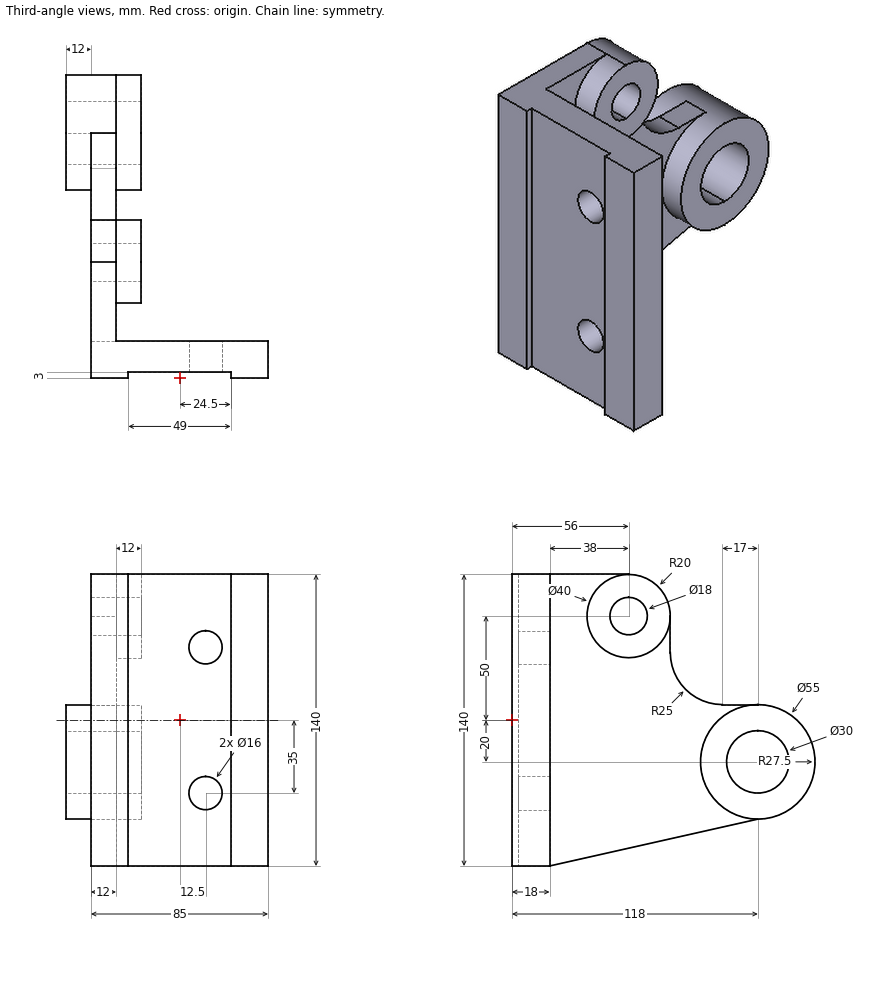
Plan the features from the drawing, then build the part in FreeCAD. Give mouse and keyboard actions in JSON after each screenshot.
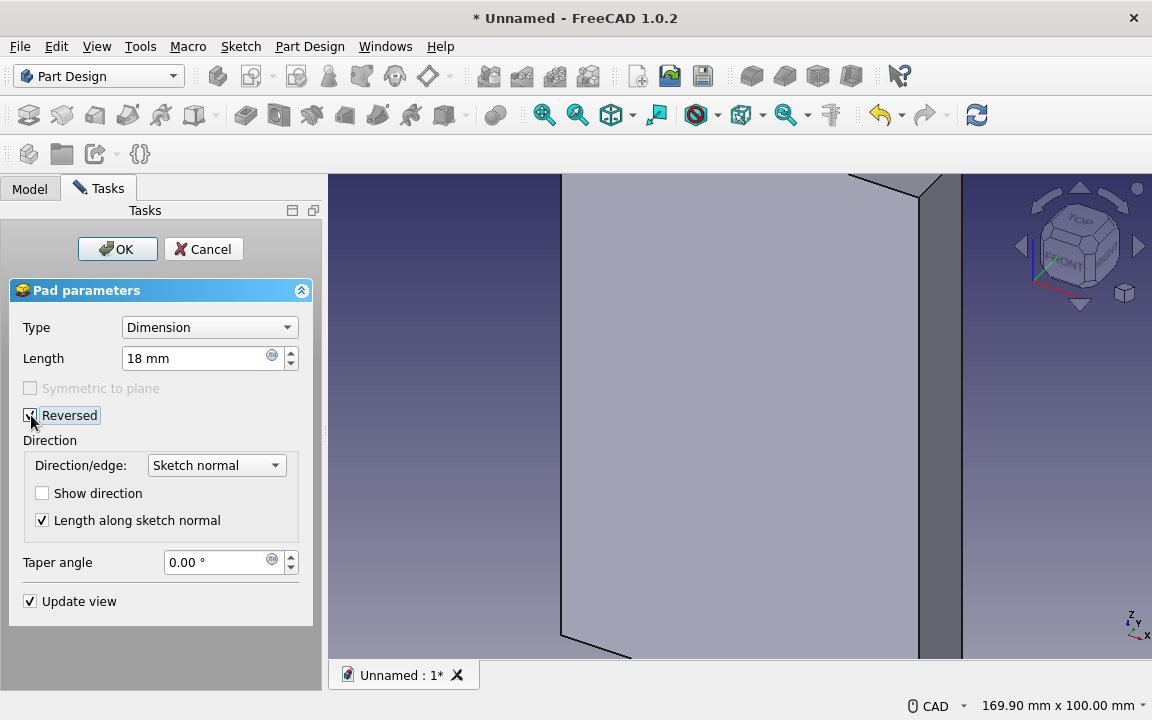
{"action": "left_click", "coordinate": [118, 249]}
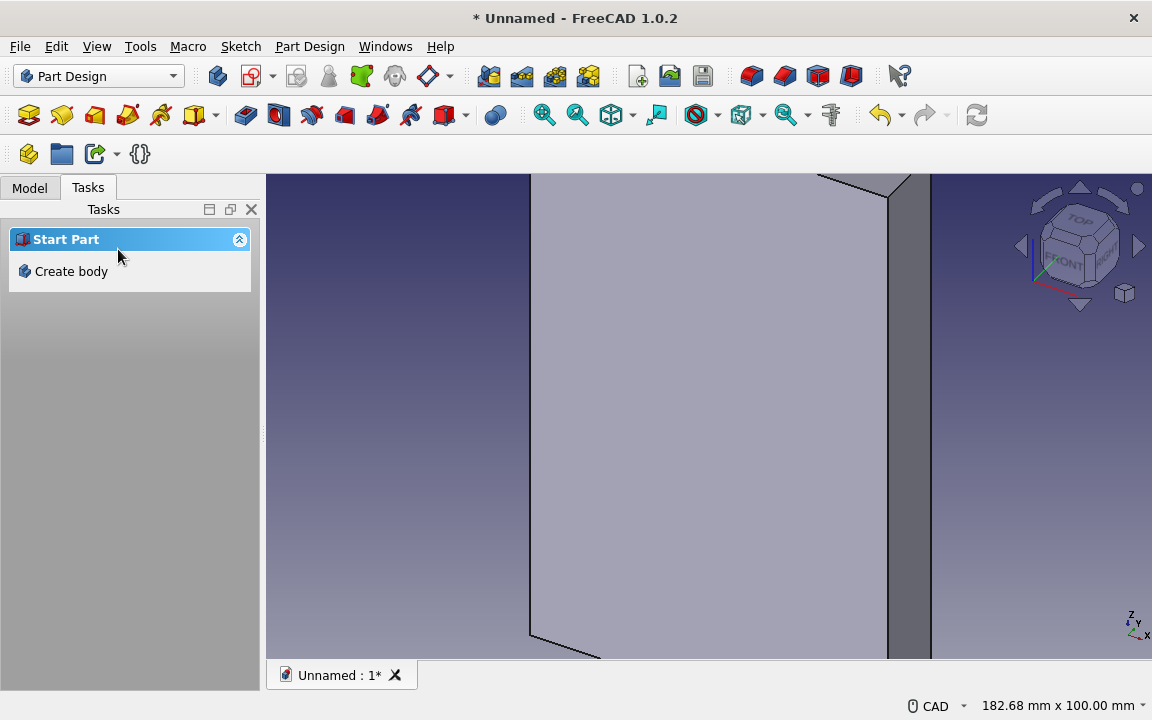
{"action": "left_click", "coordinate": [545, 116]}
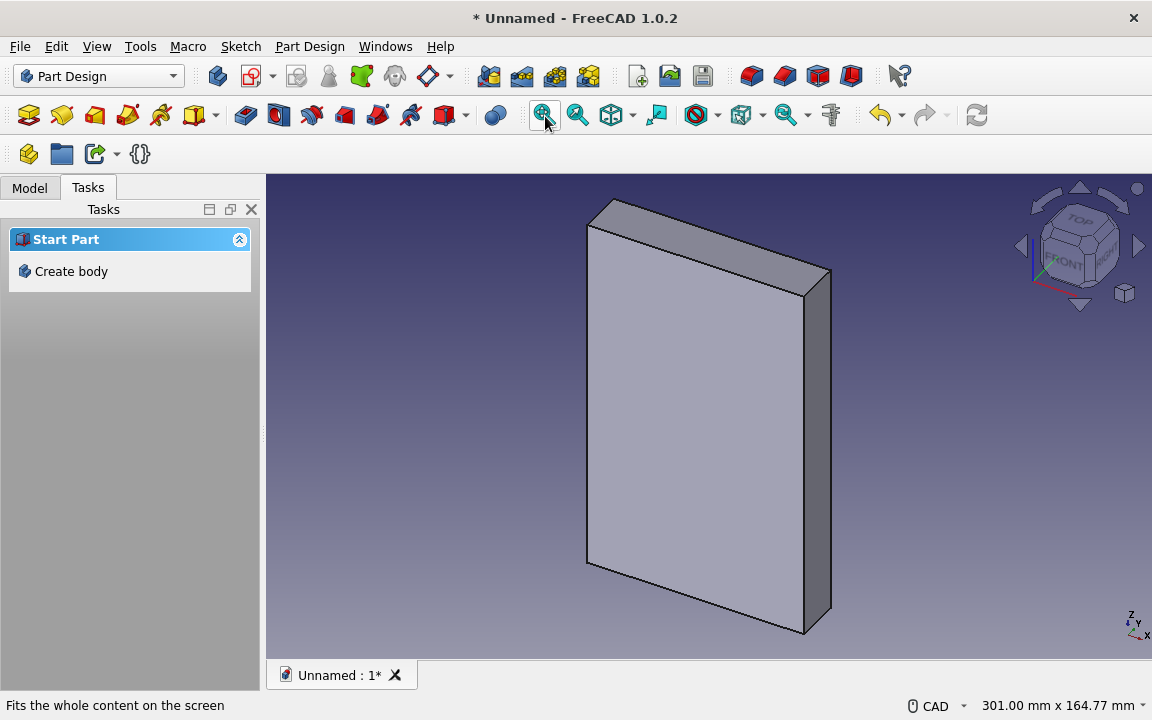
{"action": "left_click", "coordinate": [771, 267]}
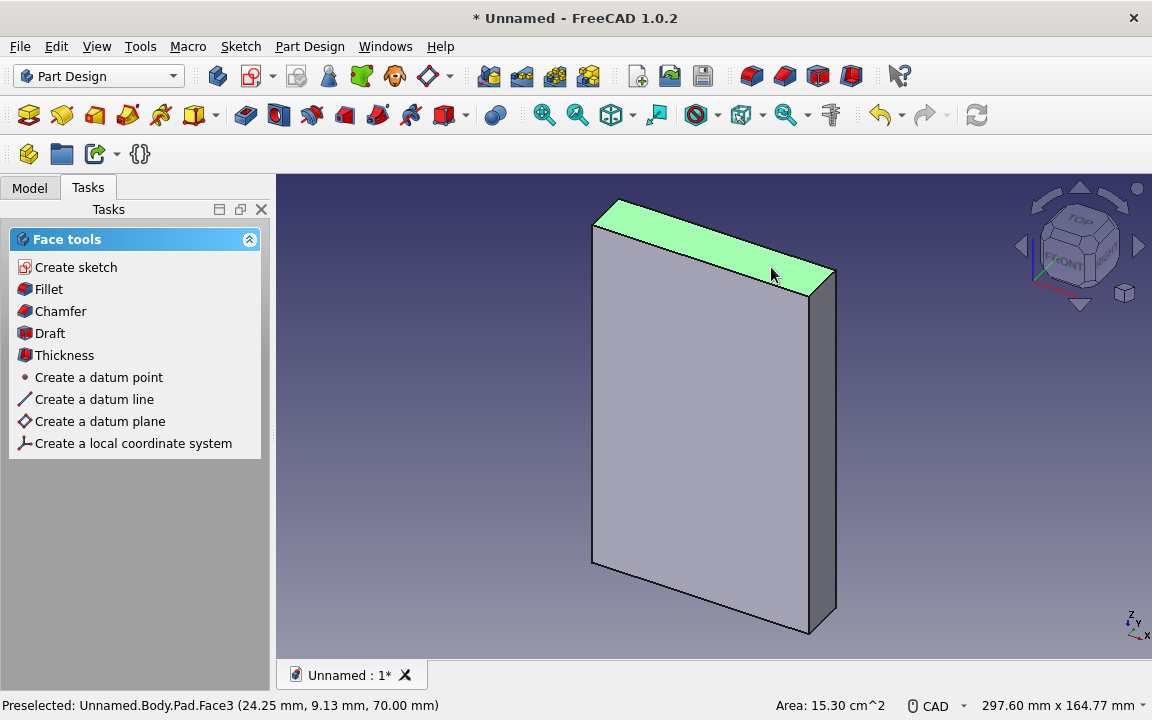
{"action": "left_click", "coordinate": [250, 76]}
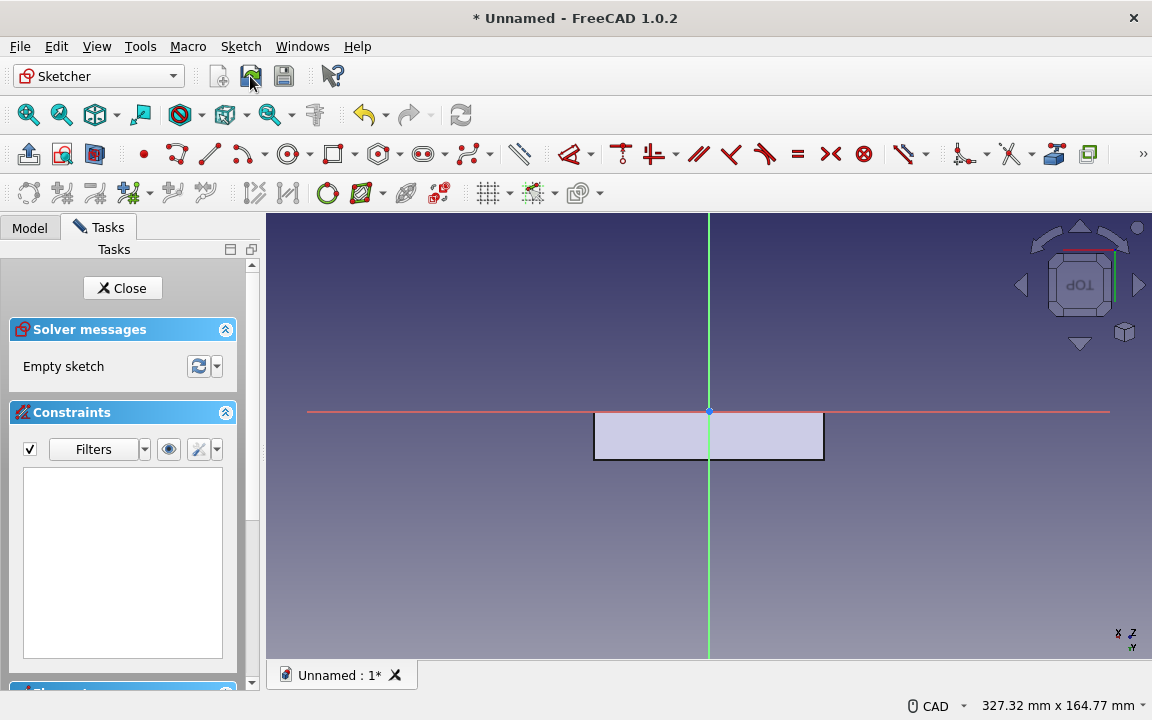
{"action": "scroll", "coordinate": [731, 409], "scroll_direction": "up", "scroll_amount": 7}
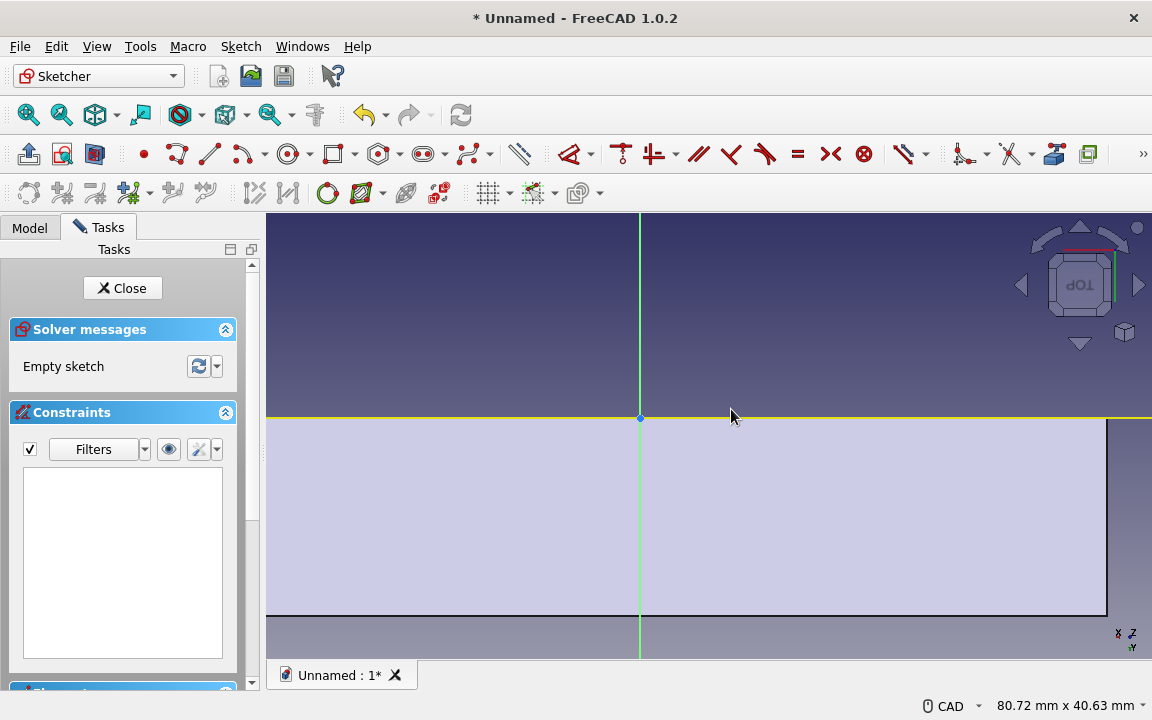
{"action": "left_click", "coordinate": [332, 154]}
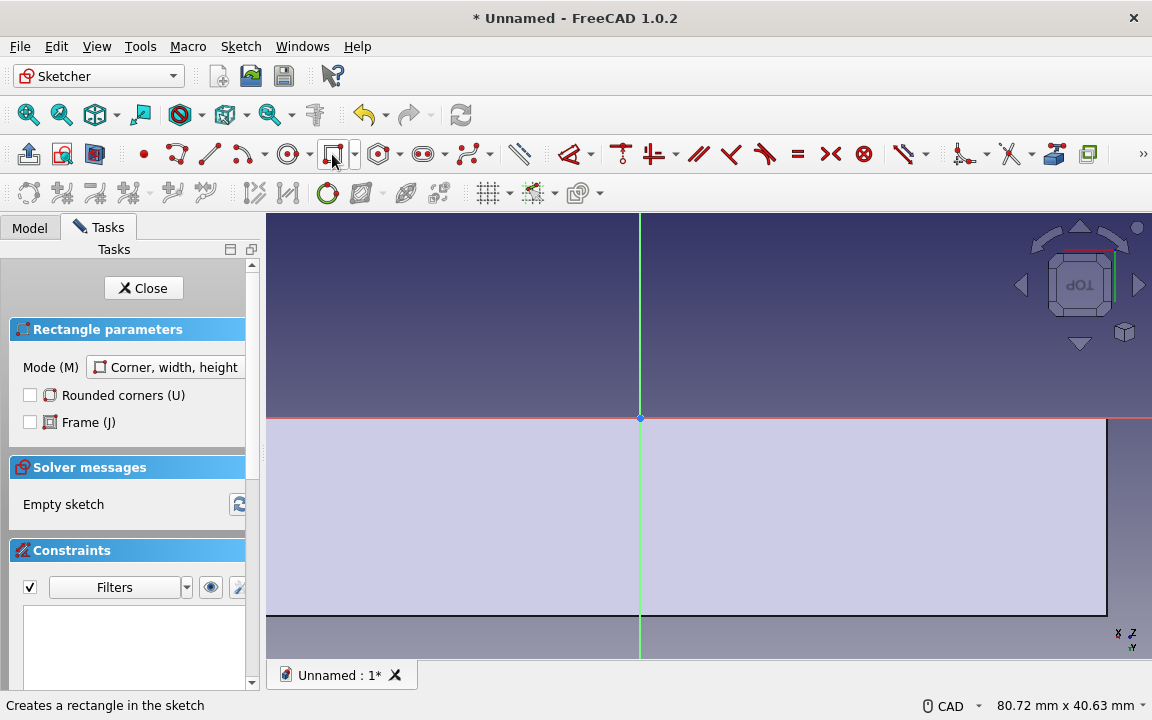
{"action": "left_click", "coordinate": [371, 418]}
{"action": "mouse_move", "coordinate": [909, 451]}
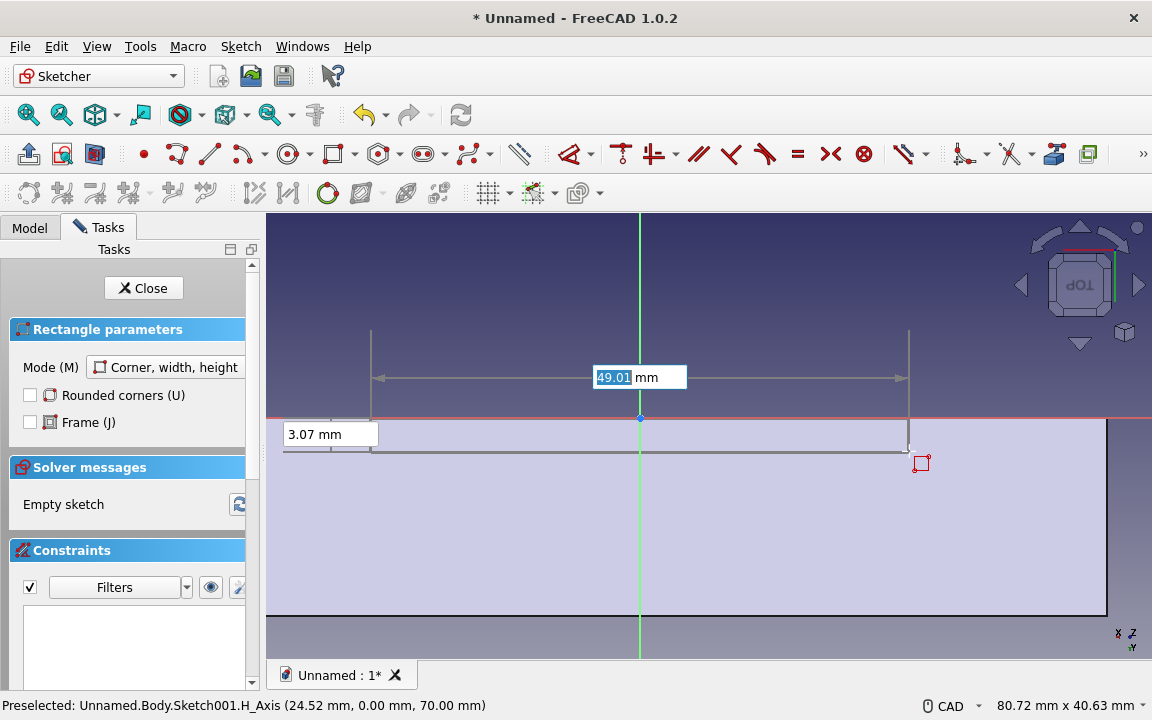
{"action": "type", "text": "49"}
{"action": "key", "text": "Tab"}
{"action": "type", "text": "3"}
{"action": "key", "text": "Return"}
{"action": "key", "text": "Escape"}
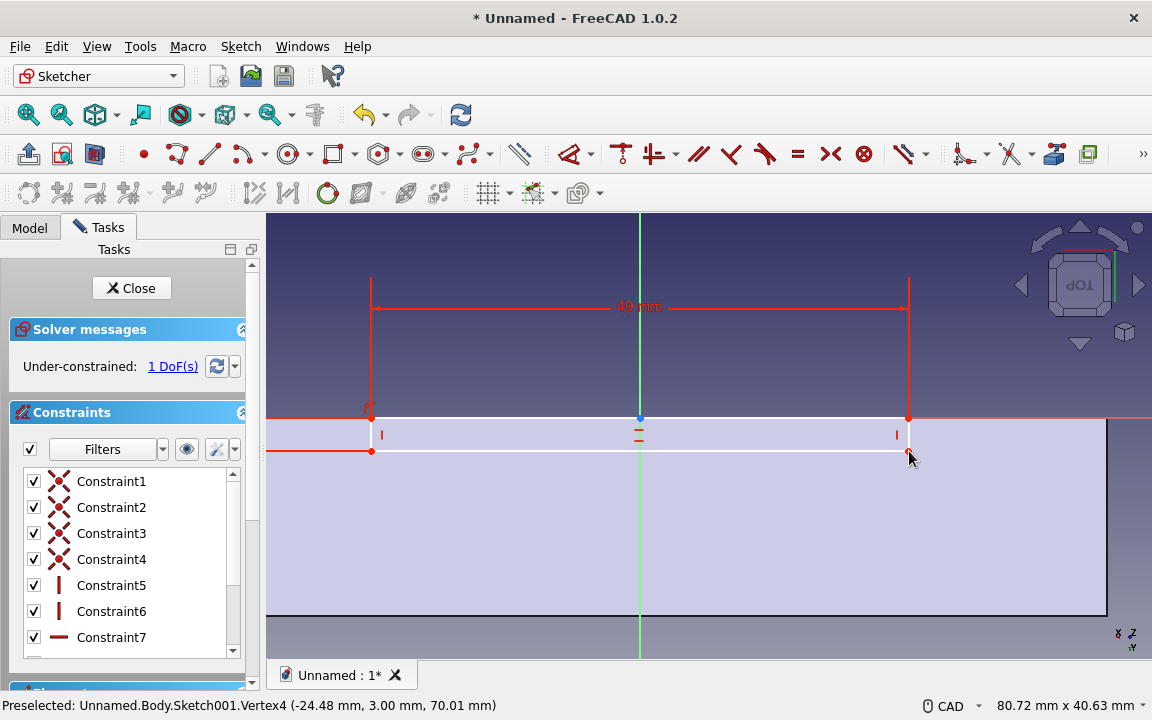
{"action": "left_click", "coordinate": [568, 154]}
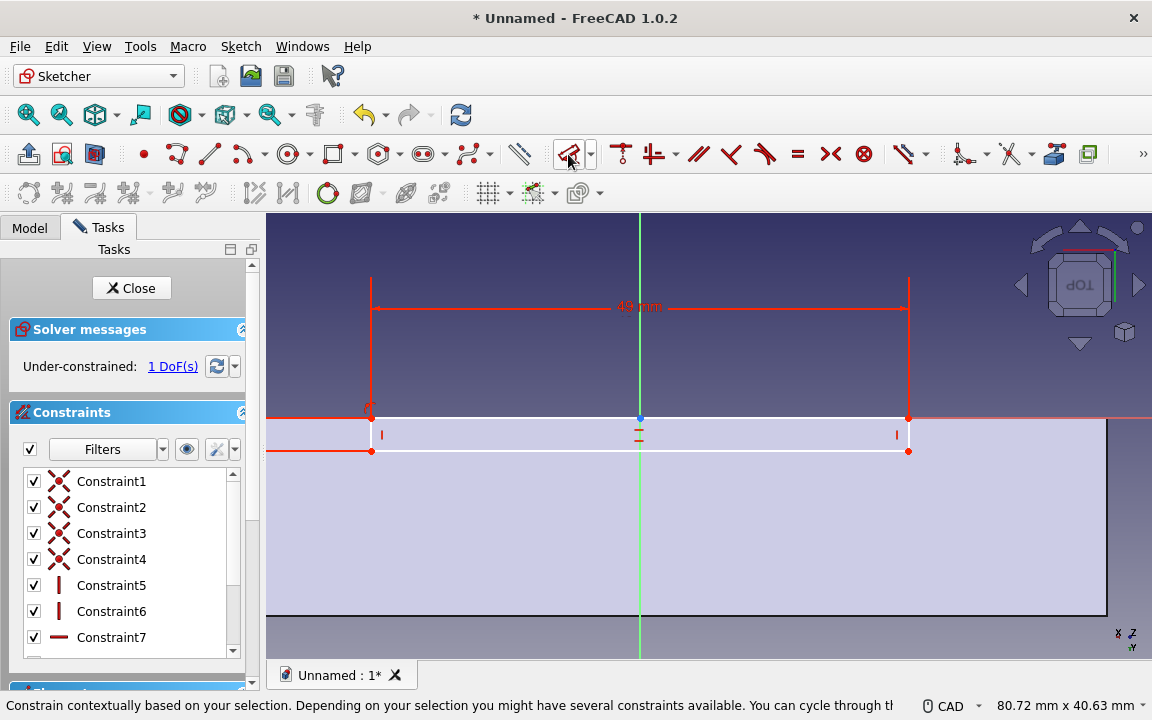
{"action": "left_click", "coordinate": [371, 418]}
{"action": "left_click", "coordinate": [506, 384]}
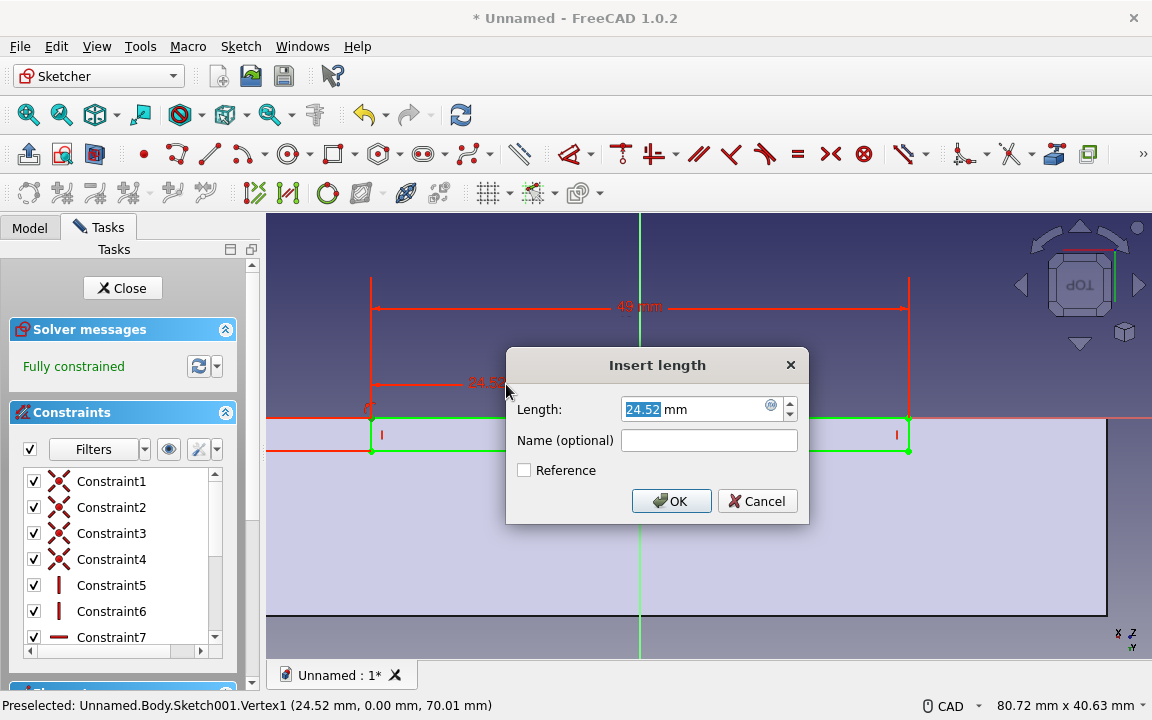
{"action": "type", "text": "24.5"}
{"action": "key", "text": "Return"}
{"action": "key", "text": "Escape"}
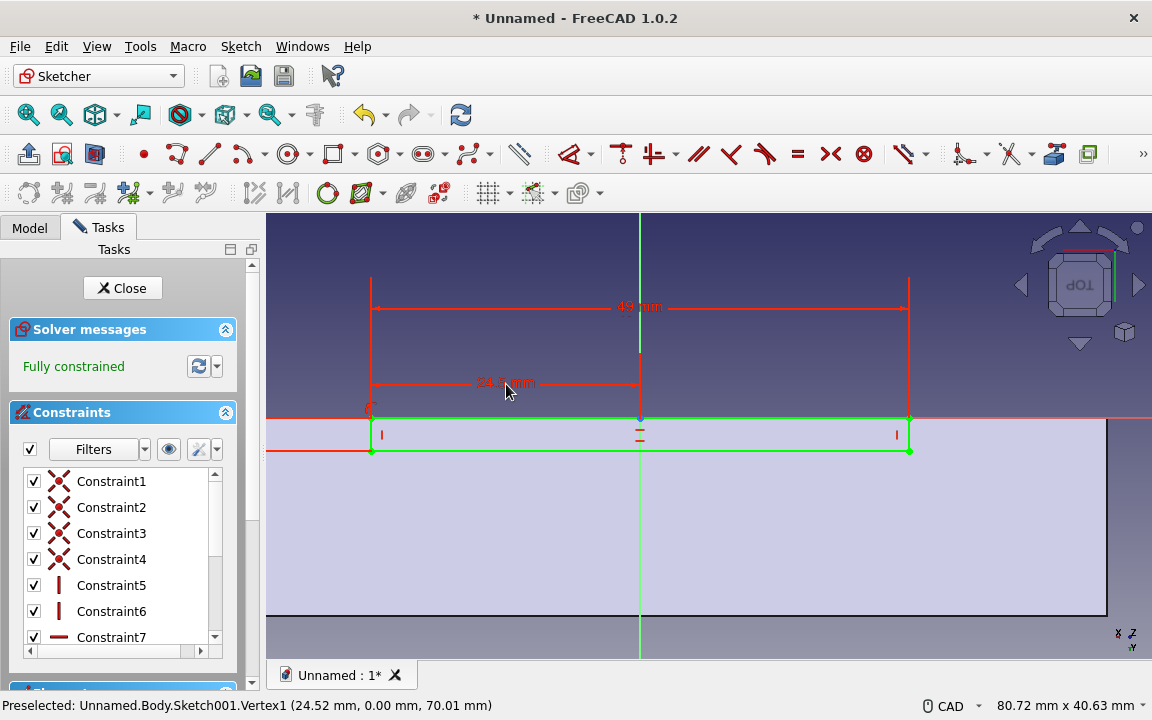
{"action": "left_click", "coordinate": [123, 288]}